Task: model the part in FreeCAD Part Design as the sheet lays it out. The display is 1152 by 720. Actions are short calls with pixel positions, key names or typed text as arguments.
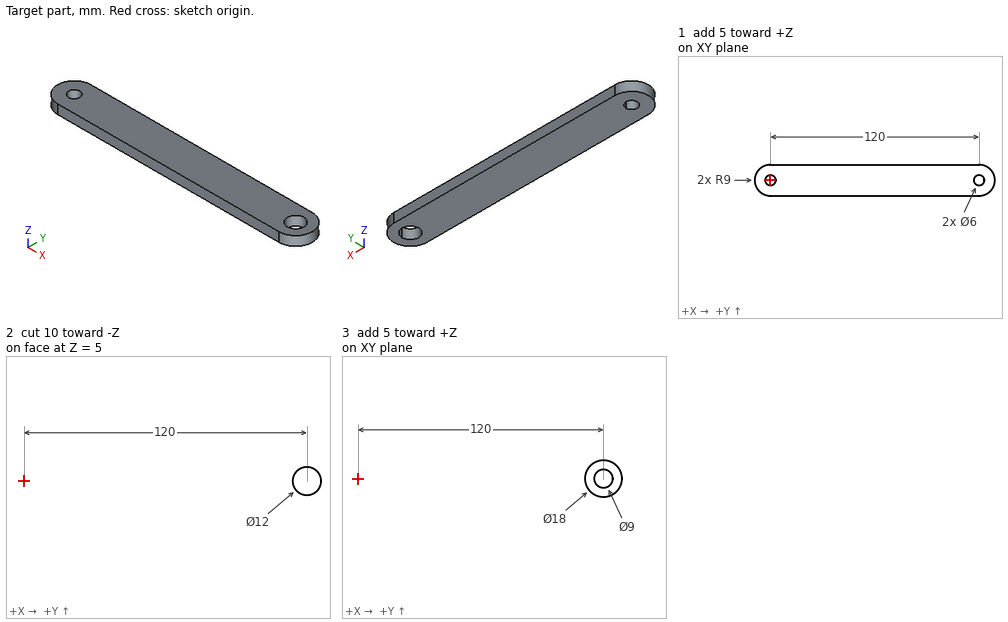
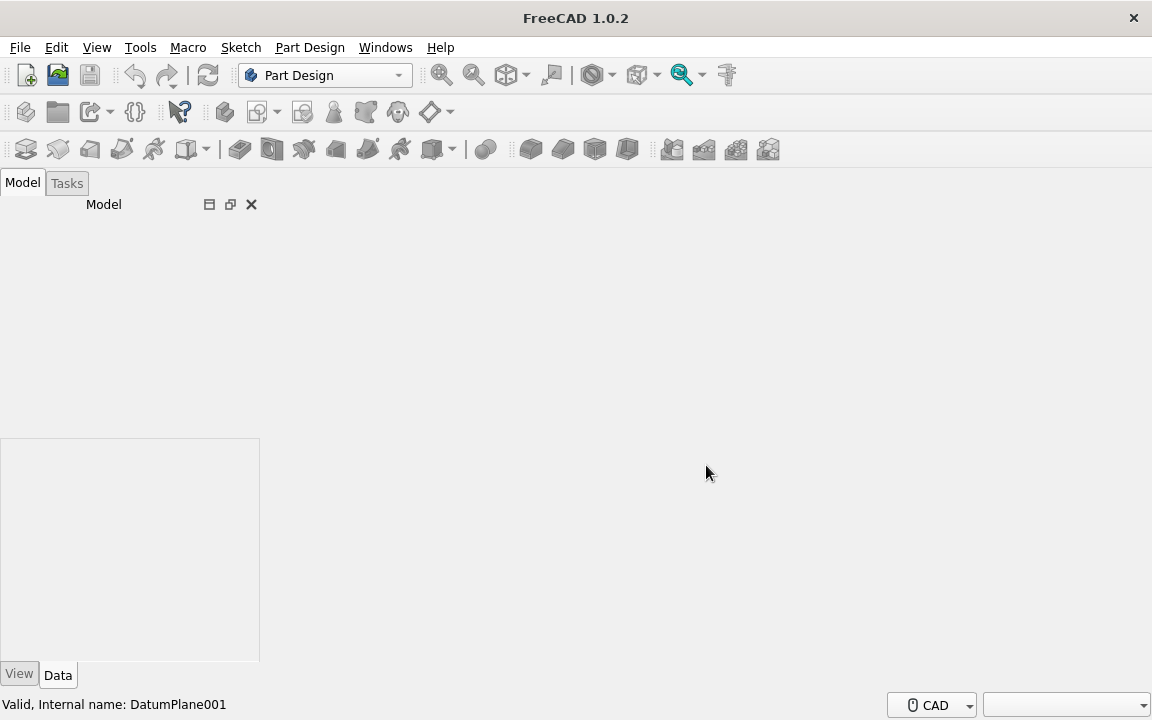
click(26, 76)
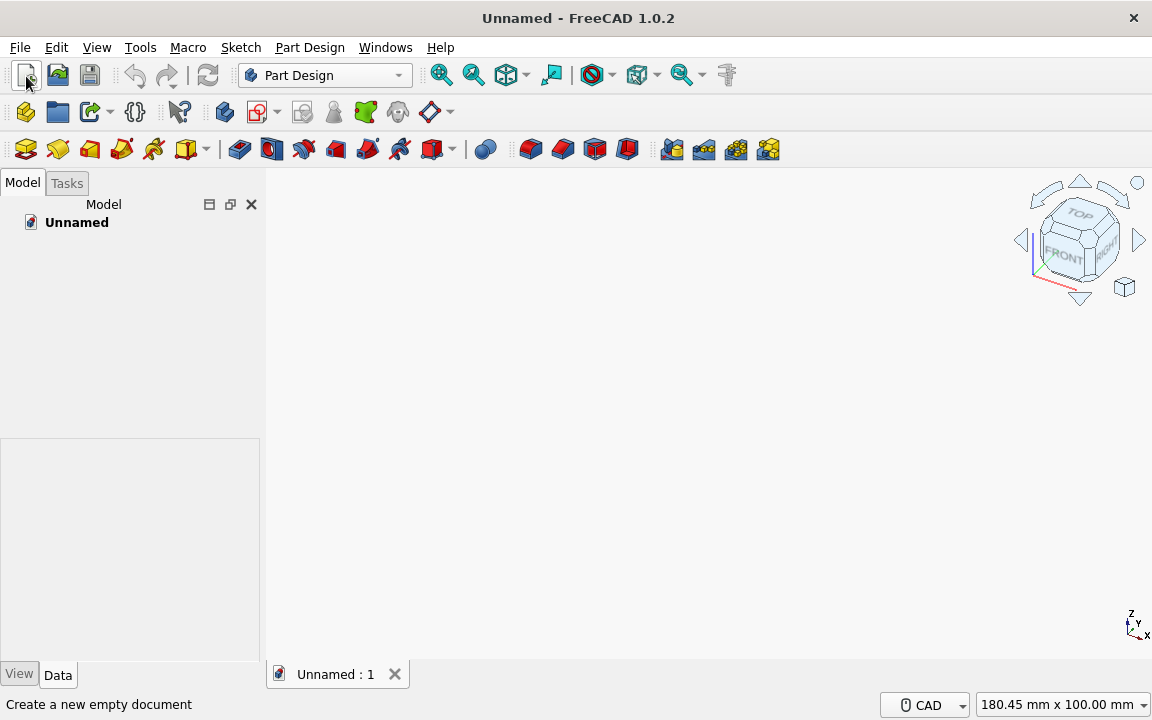
click(258, 112)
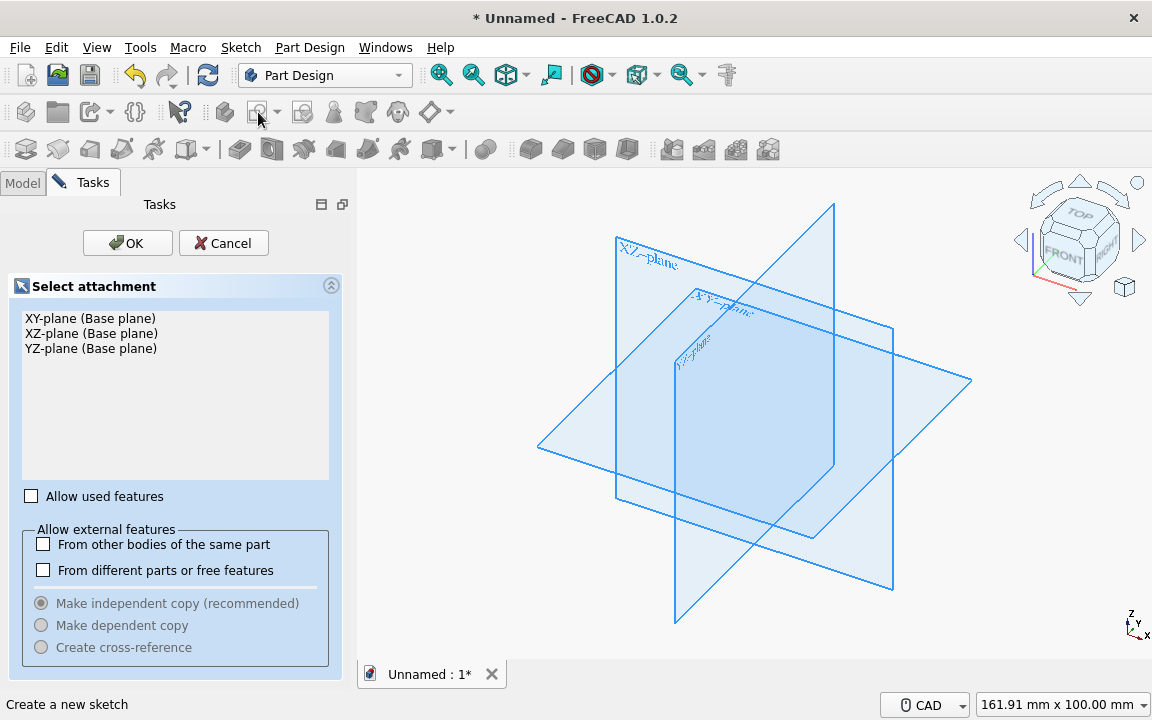
click(82, 318)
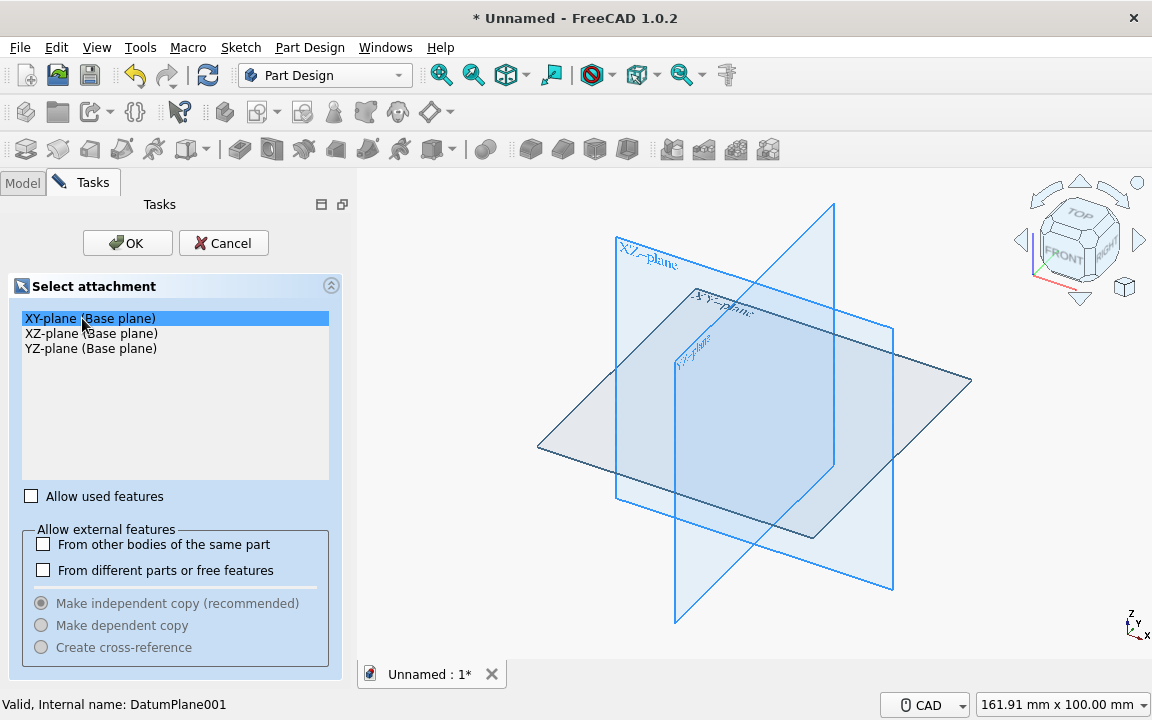
click(128, 243)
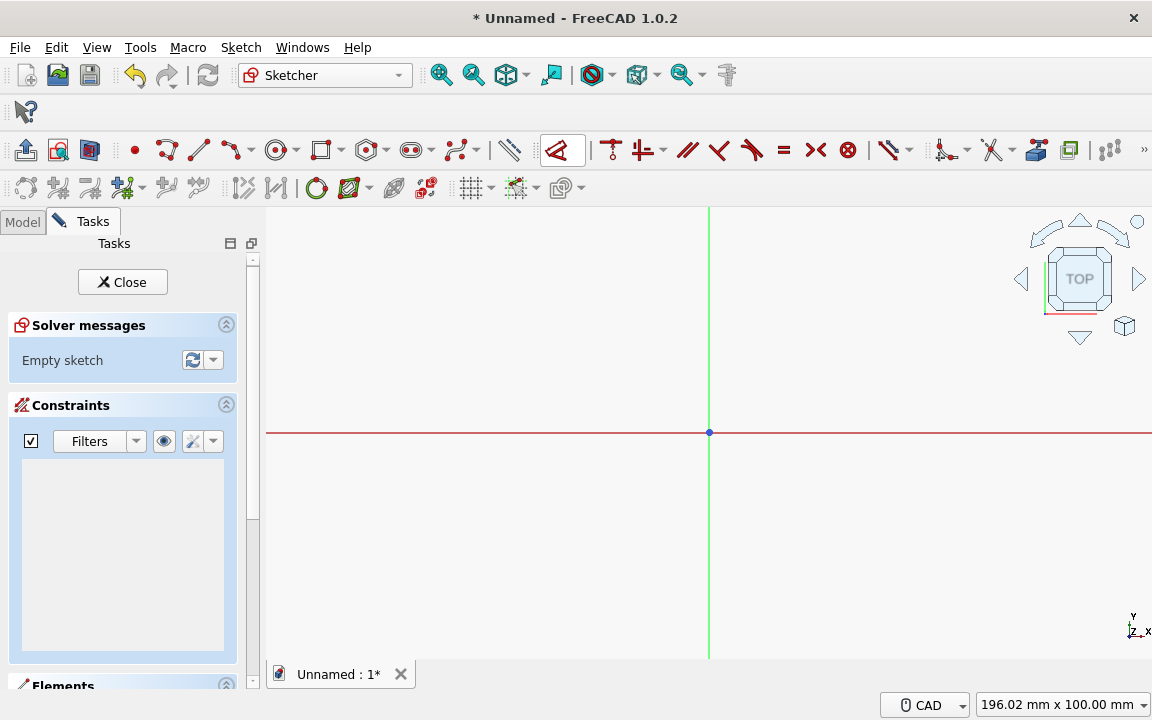
scroll(294, 433, down, 3)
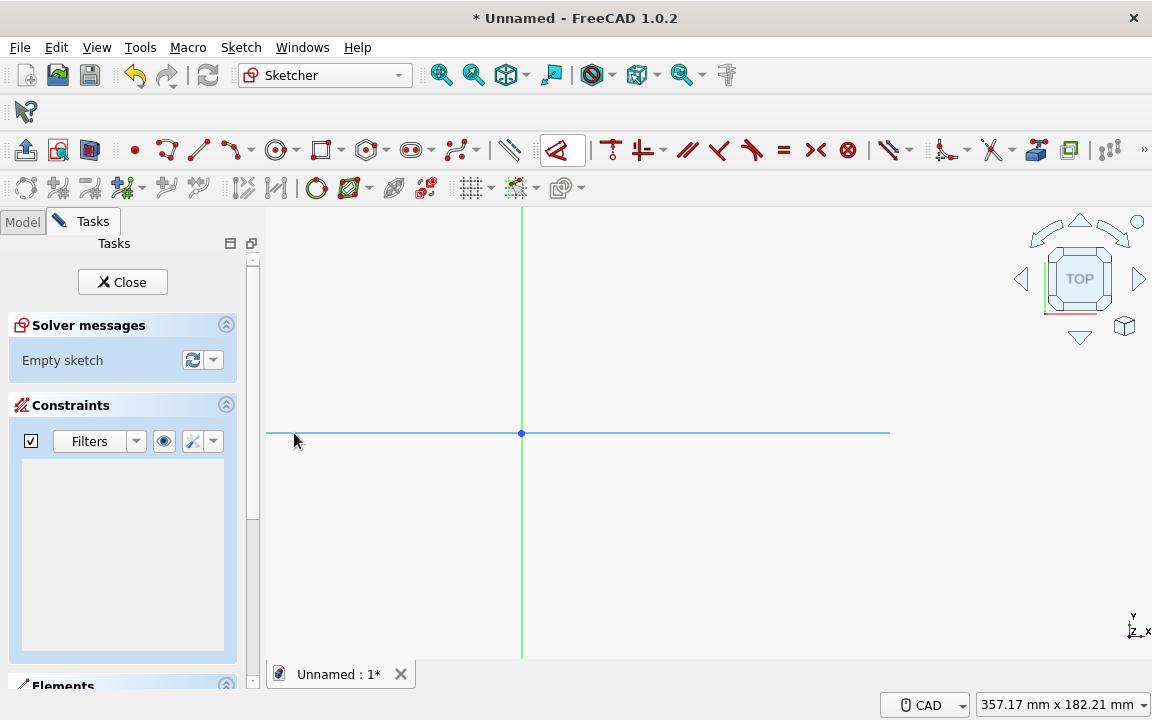
scroll(732, 434, up, 2)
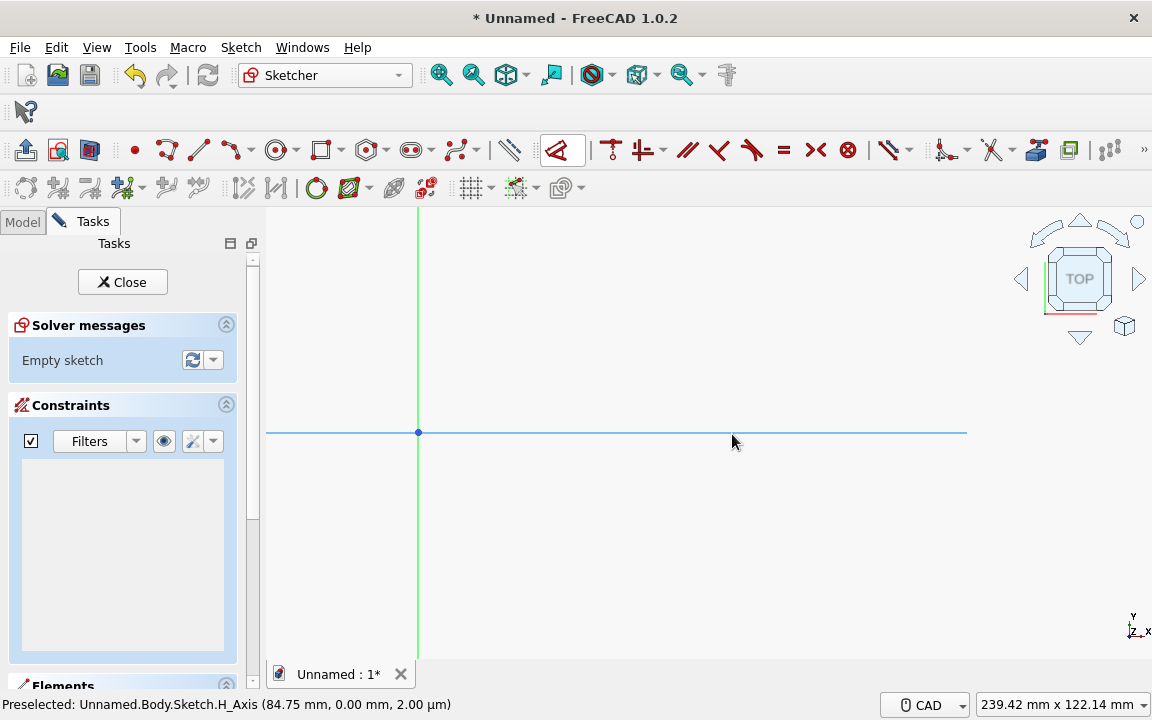
click(412, 150)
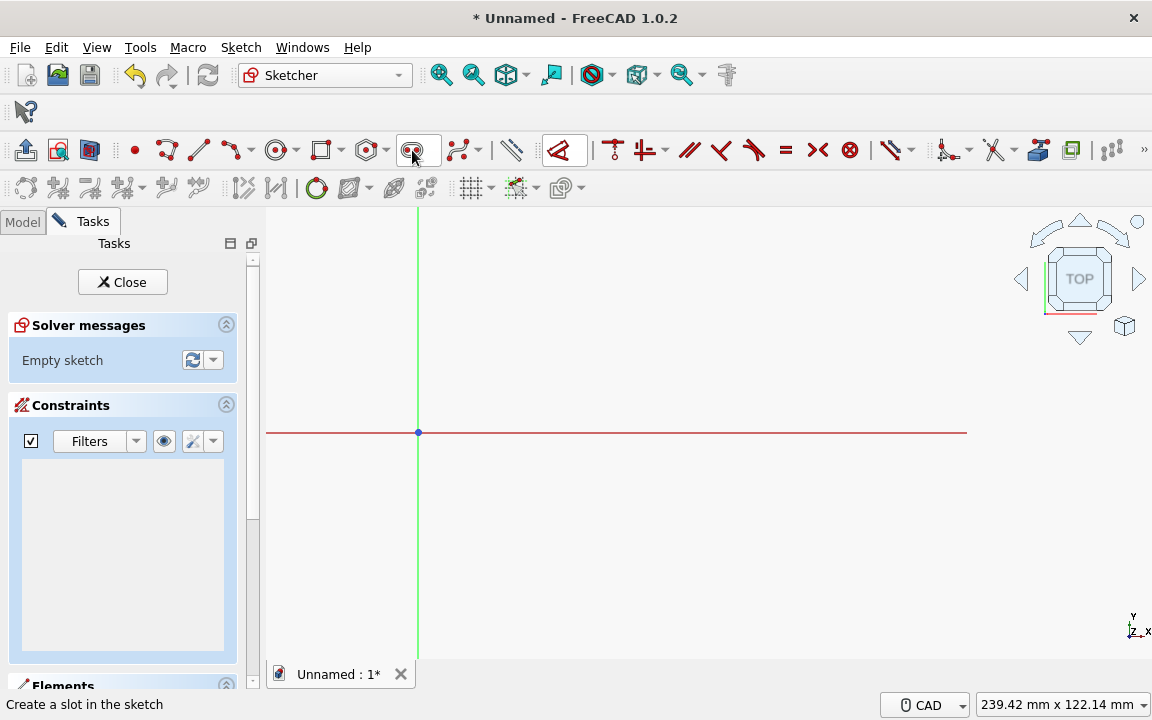
click(418, 433)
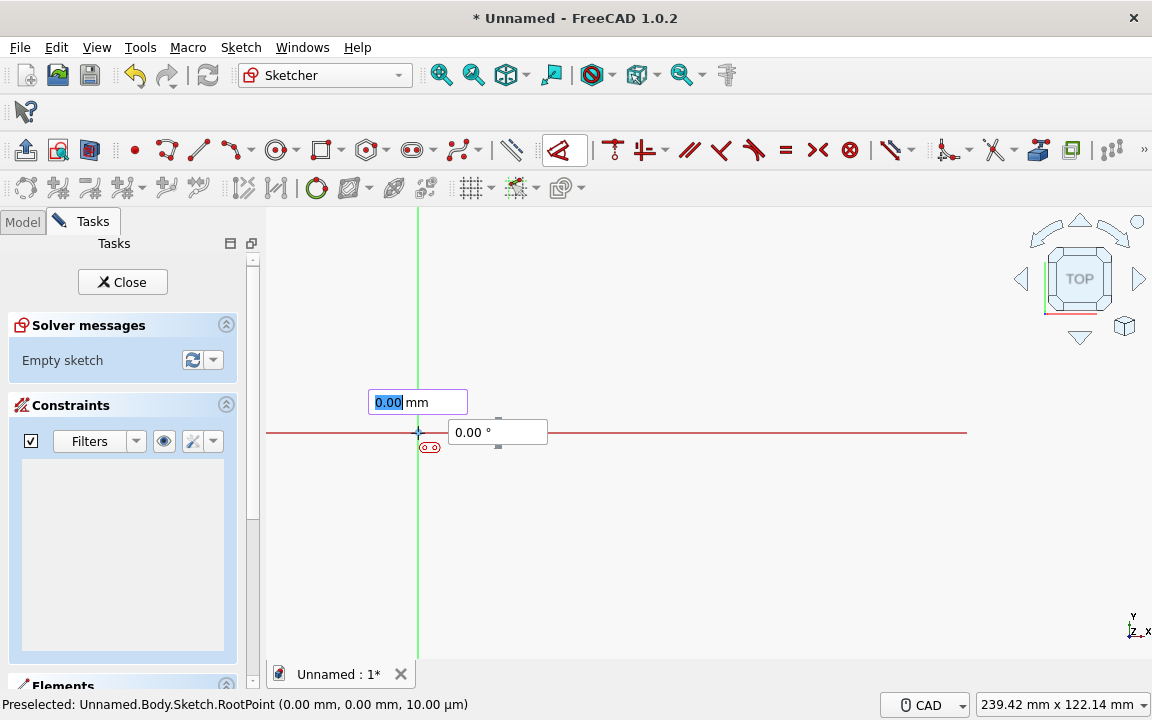
click(862, 424)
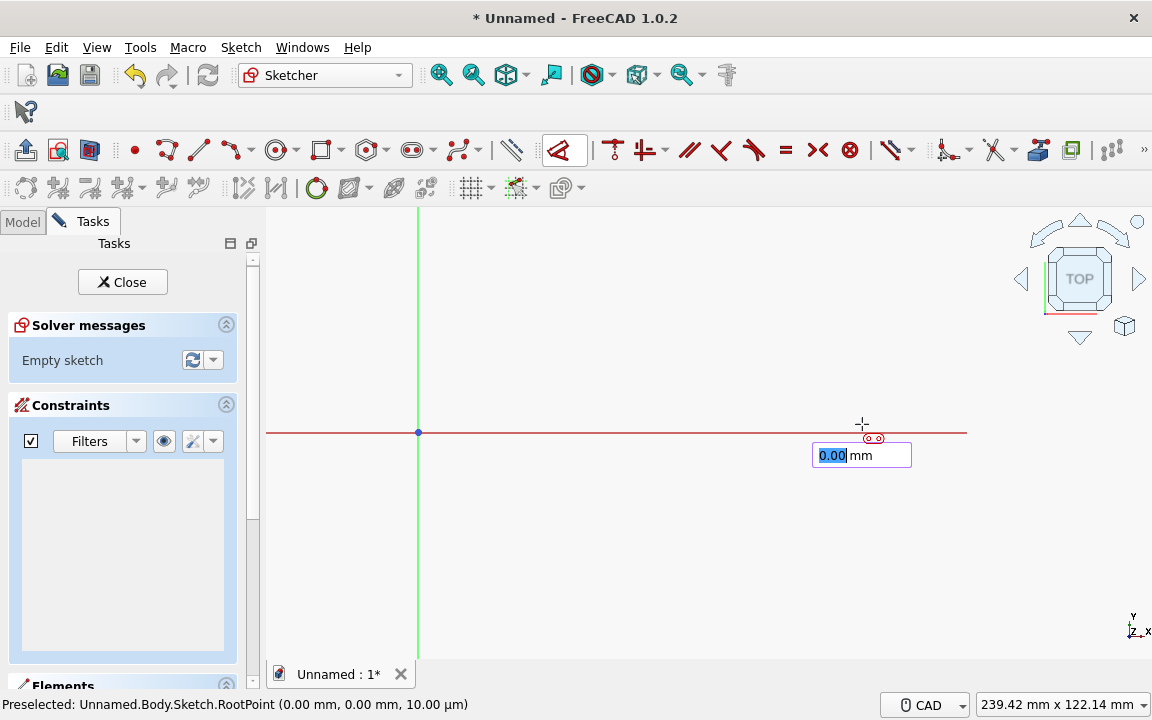
click(640, 399)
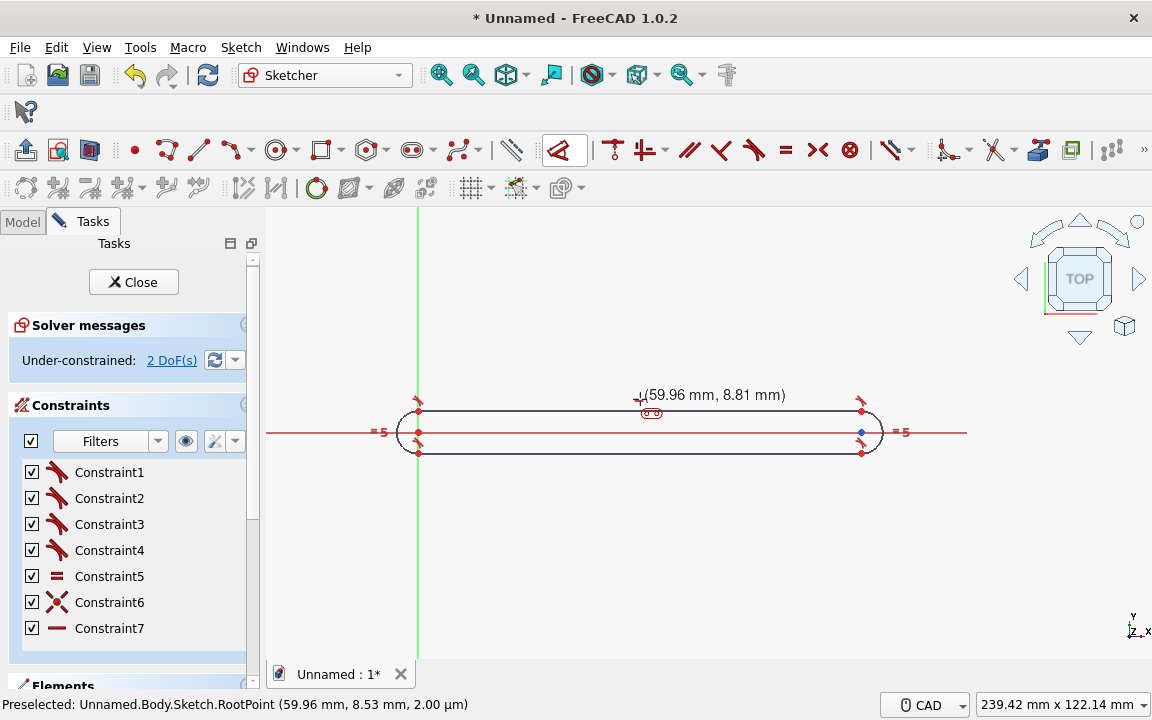
click(276, 150)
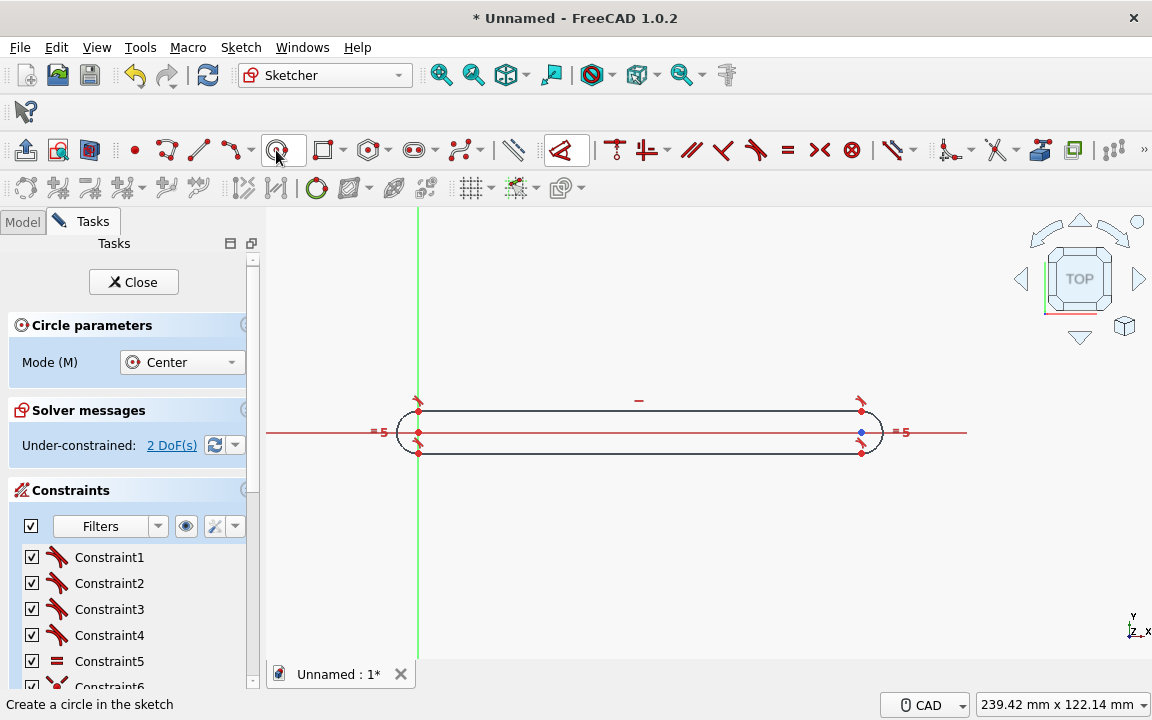
scroll(862, 433, up, 4)